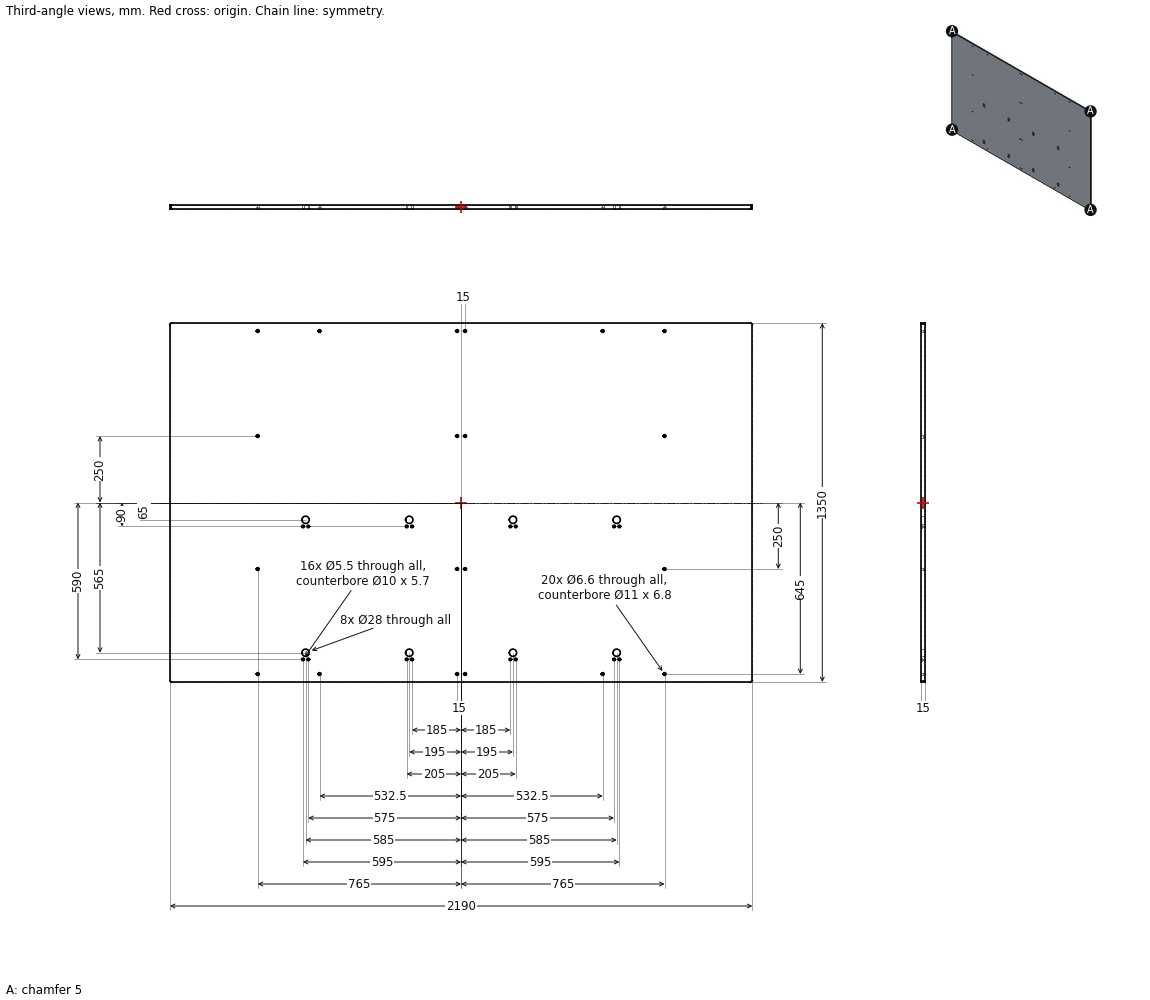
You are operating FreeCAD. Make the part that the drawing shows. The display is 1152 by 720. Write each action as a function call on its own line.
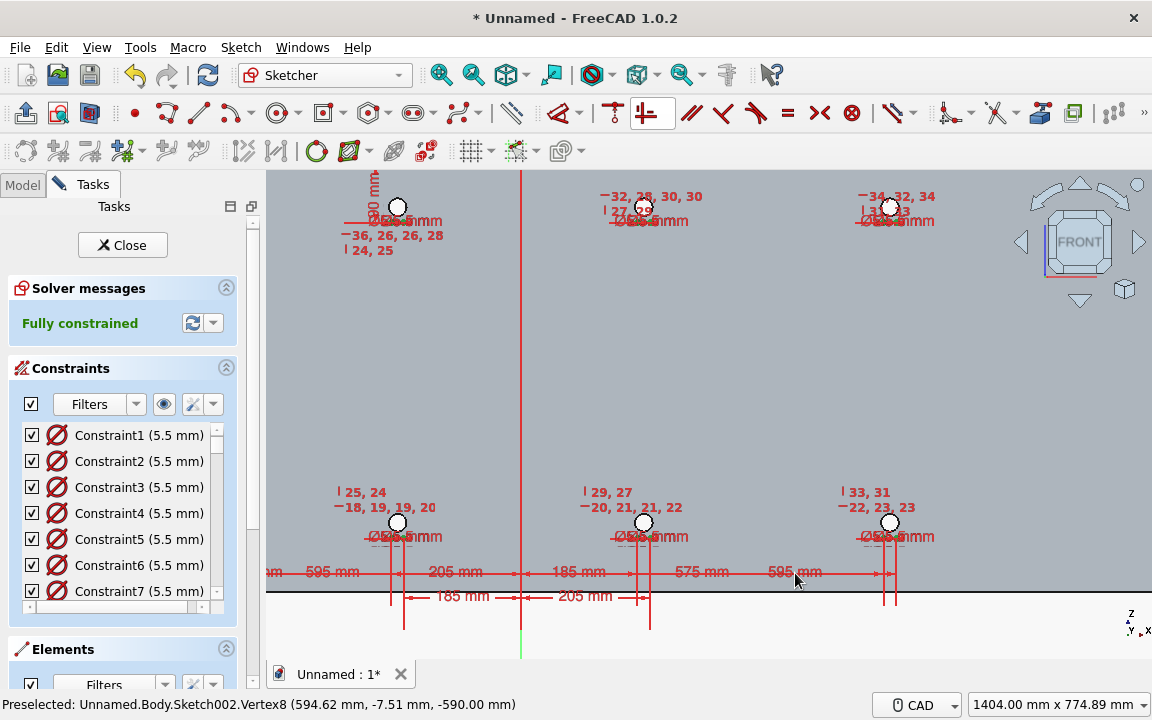
click(123, 245)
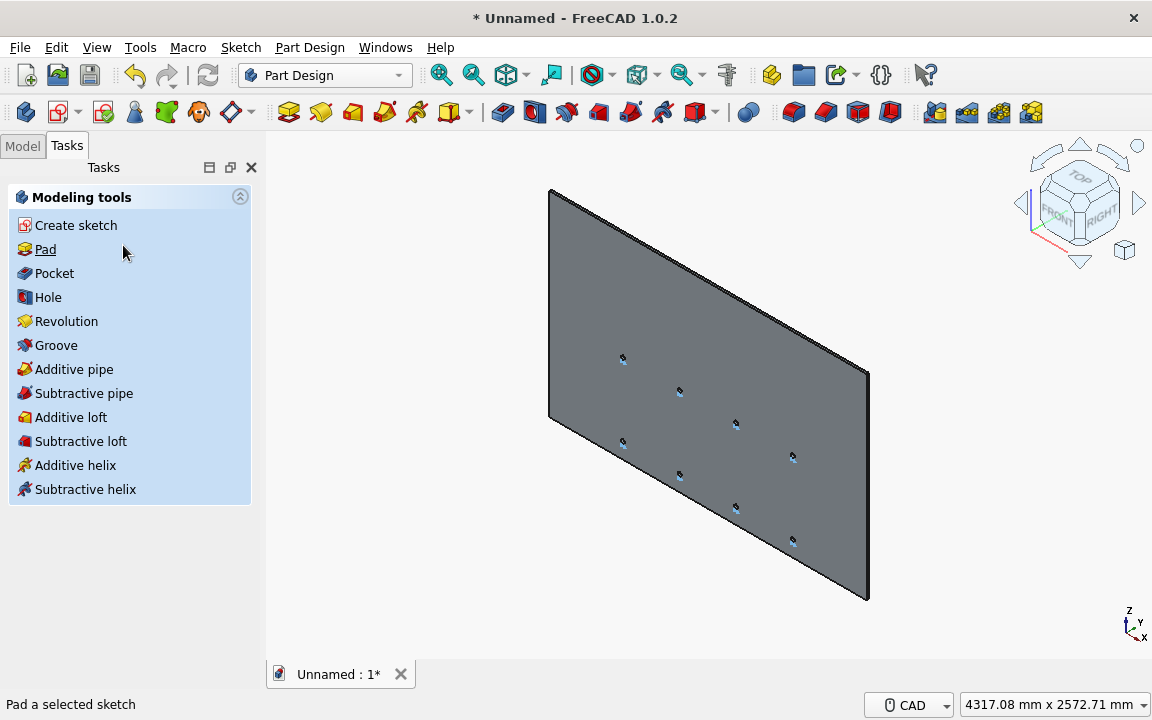
click(536, 112)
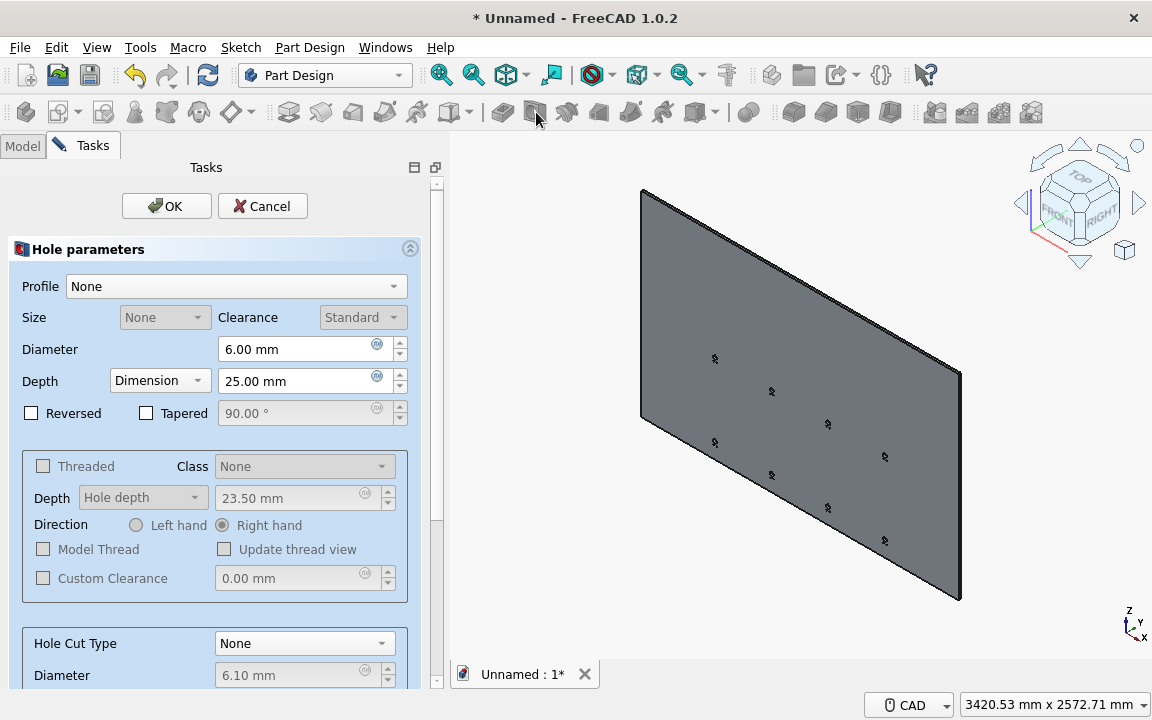
triple_click(305, 349)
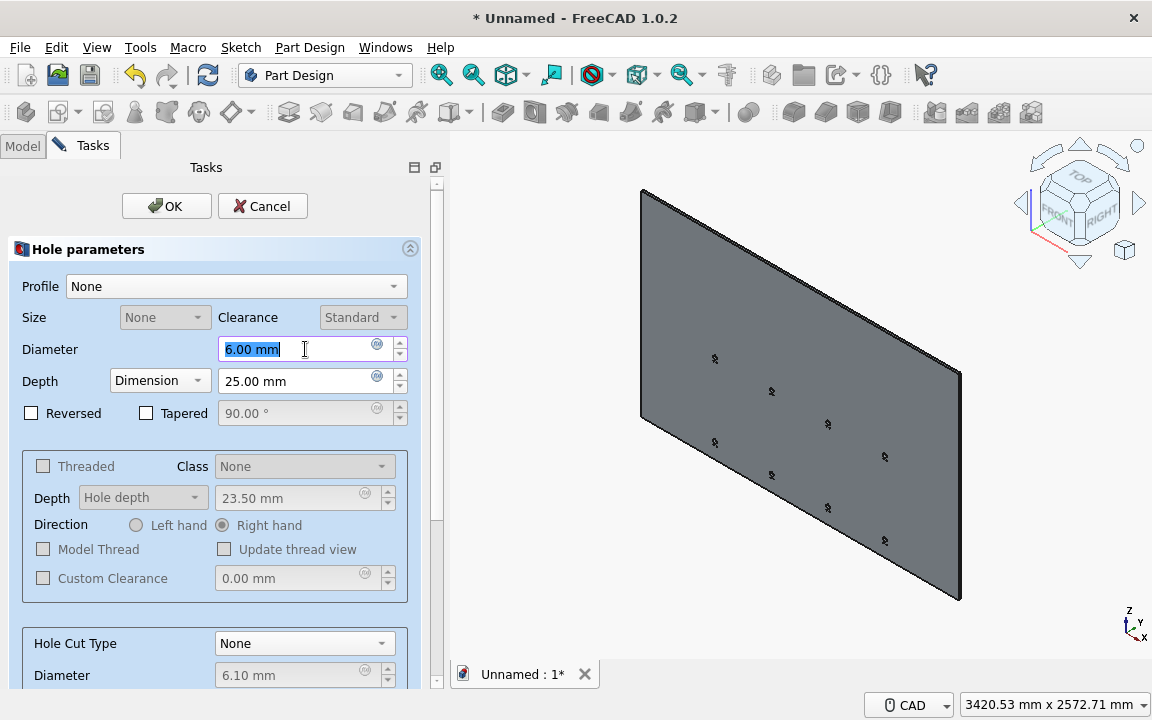
text(5.5)
key(Tab)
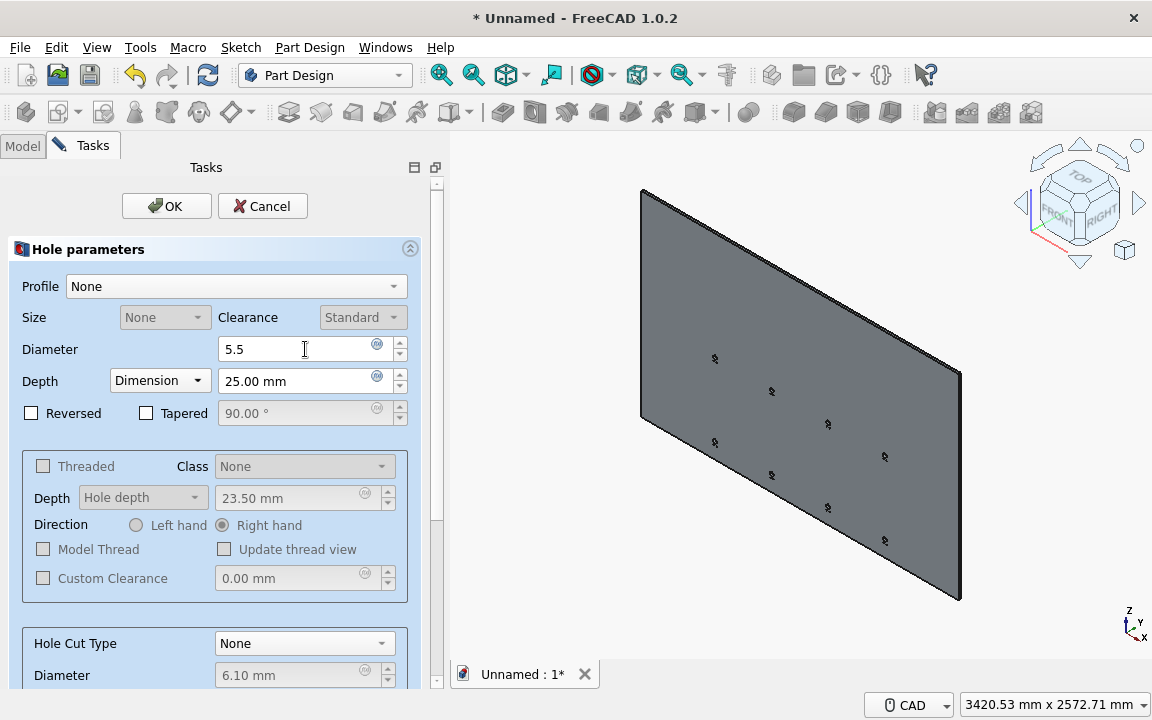
click(161, 380)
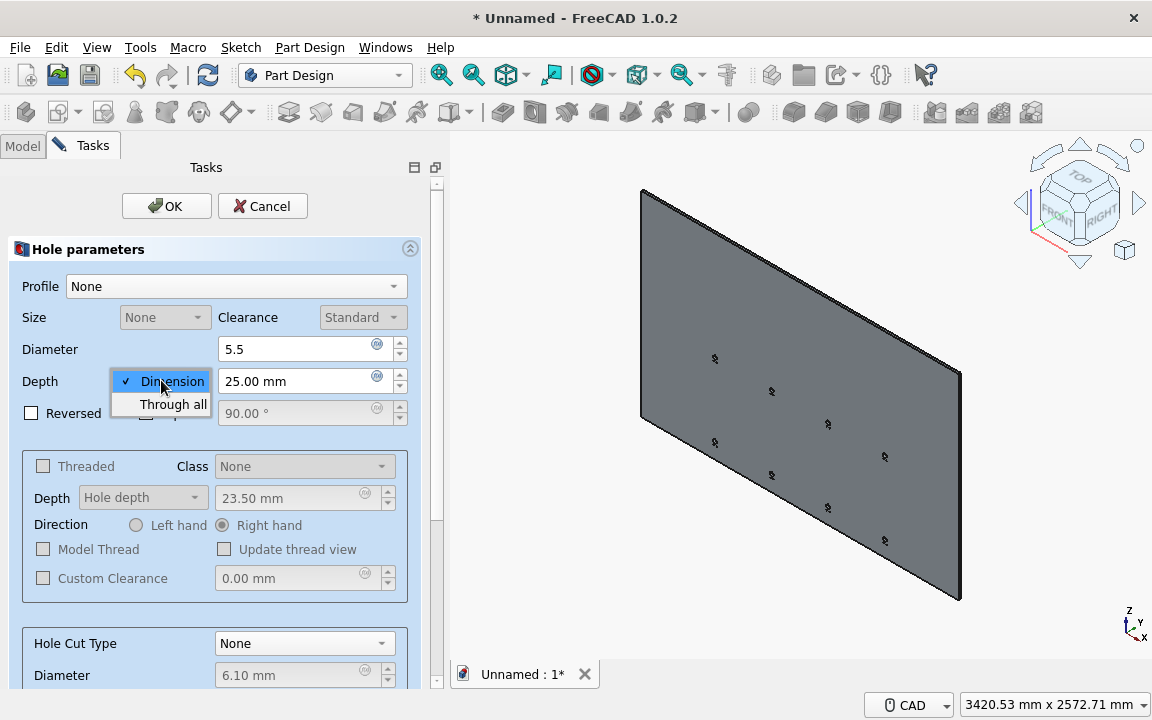
click(160, 404)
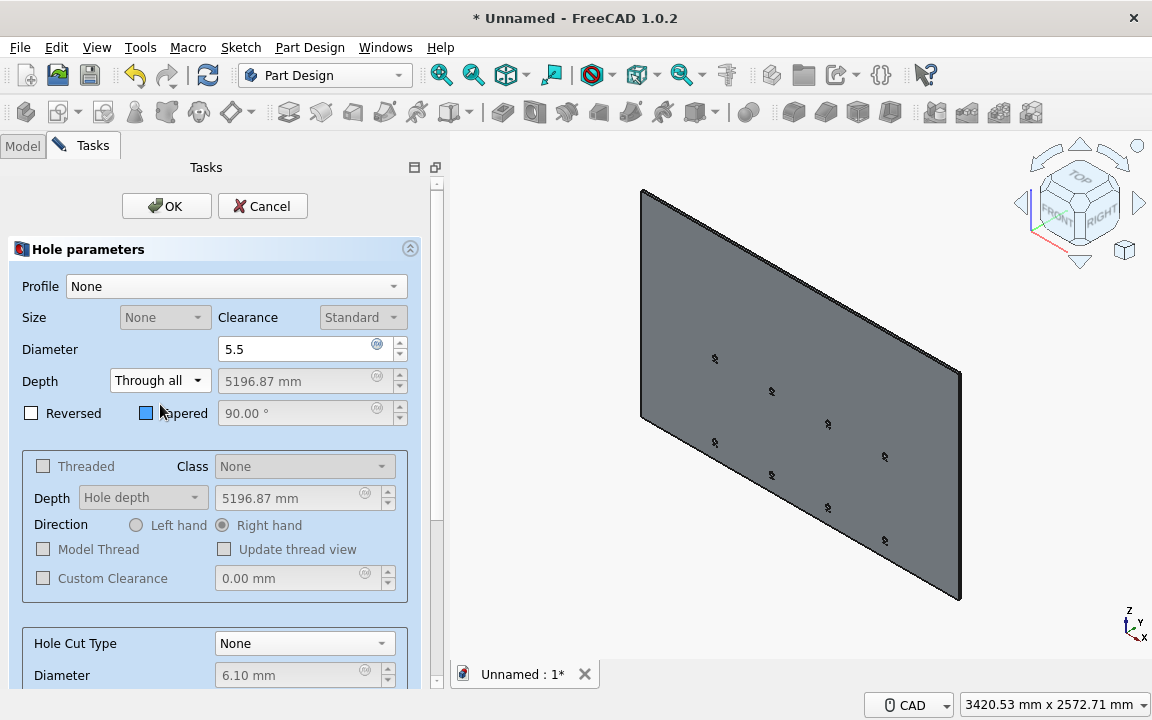
click(306, 644)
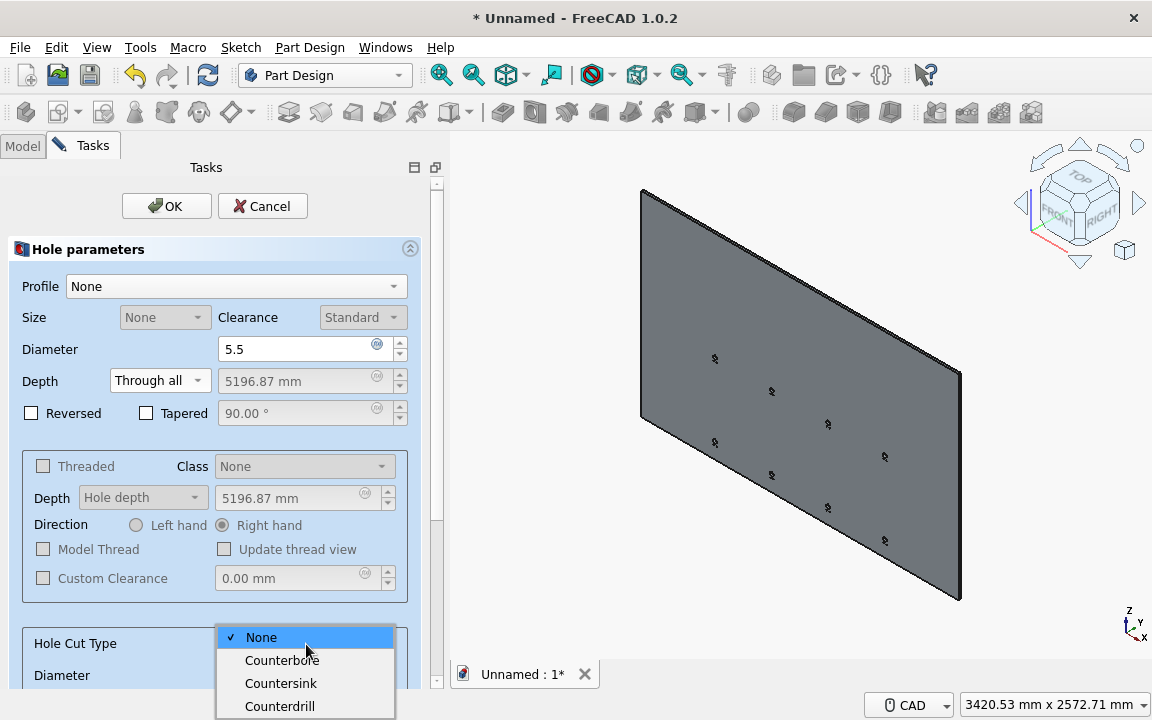
click(304, 660)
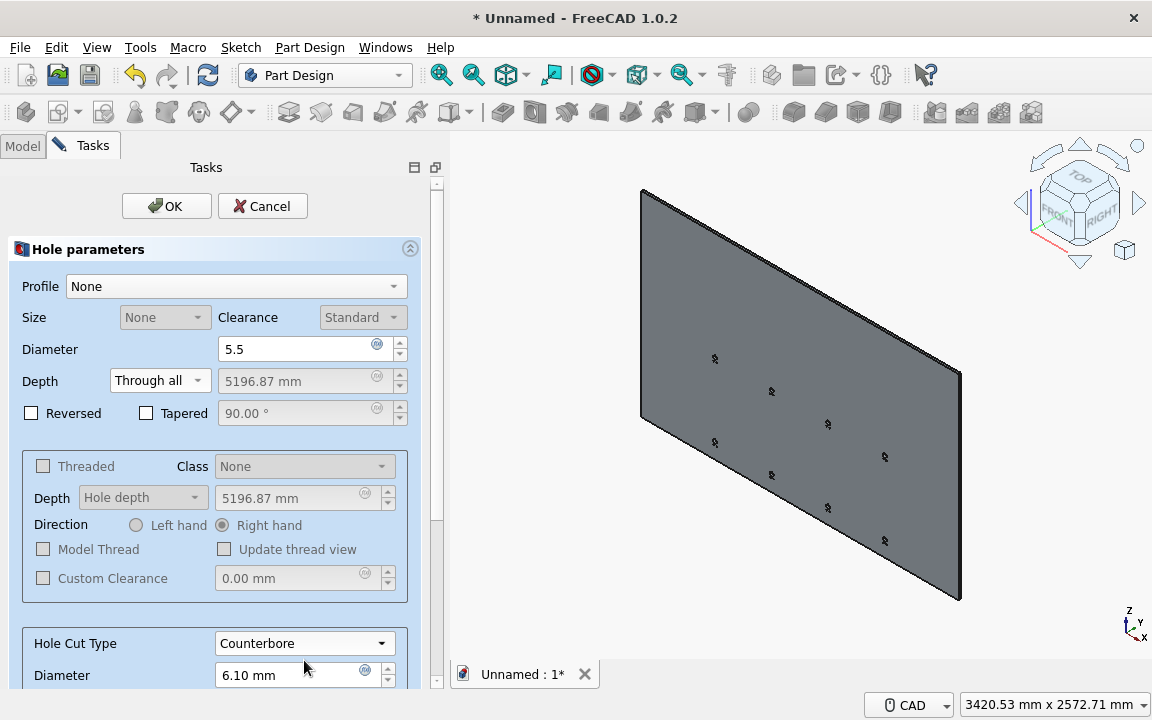
triple_click(298, 675)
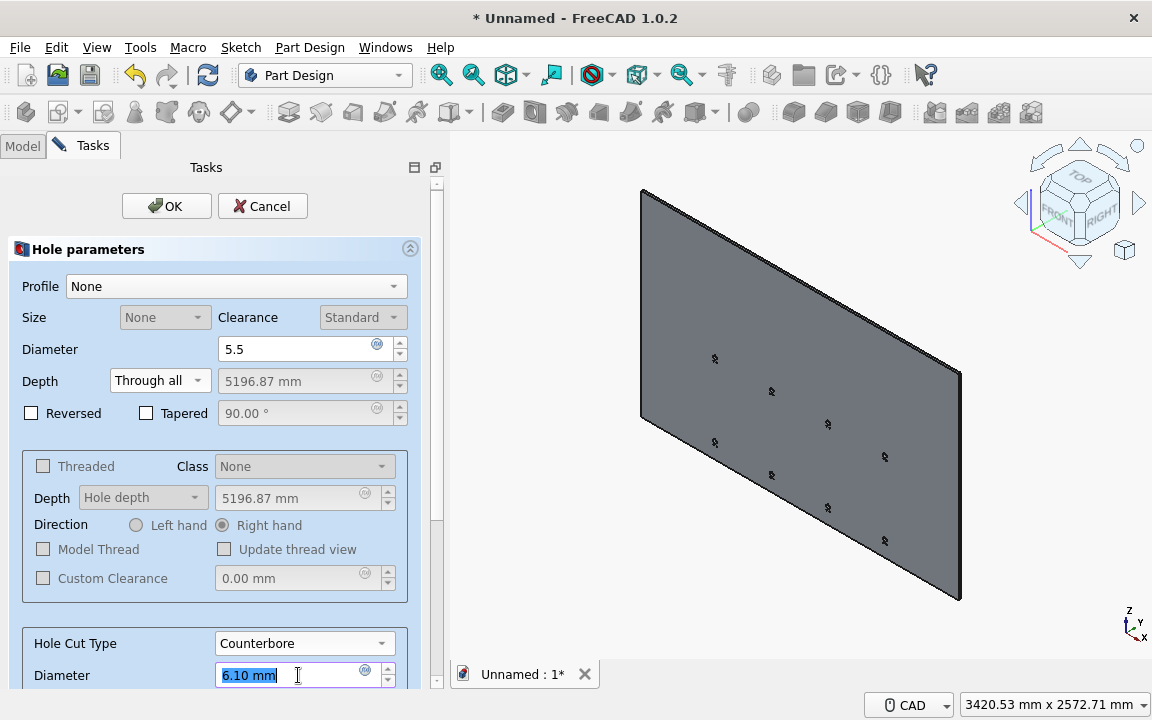
text(10)
key(Tab)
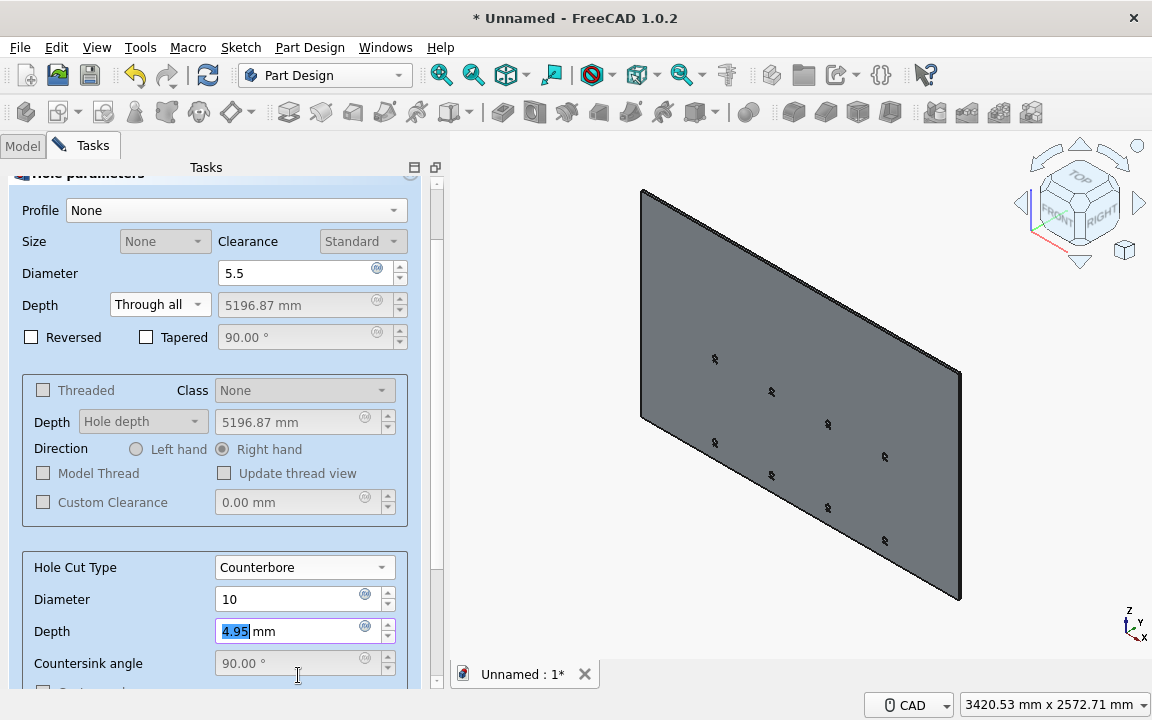
text(5.7)
key(Tab)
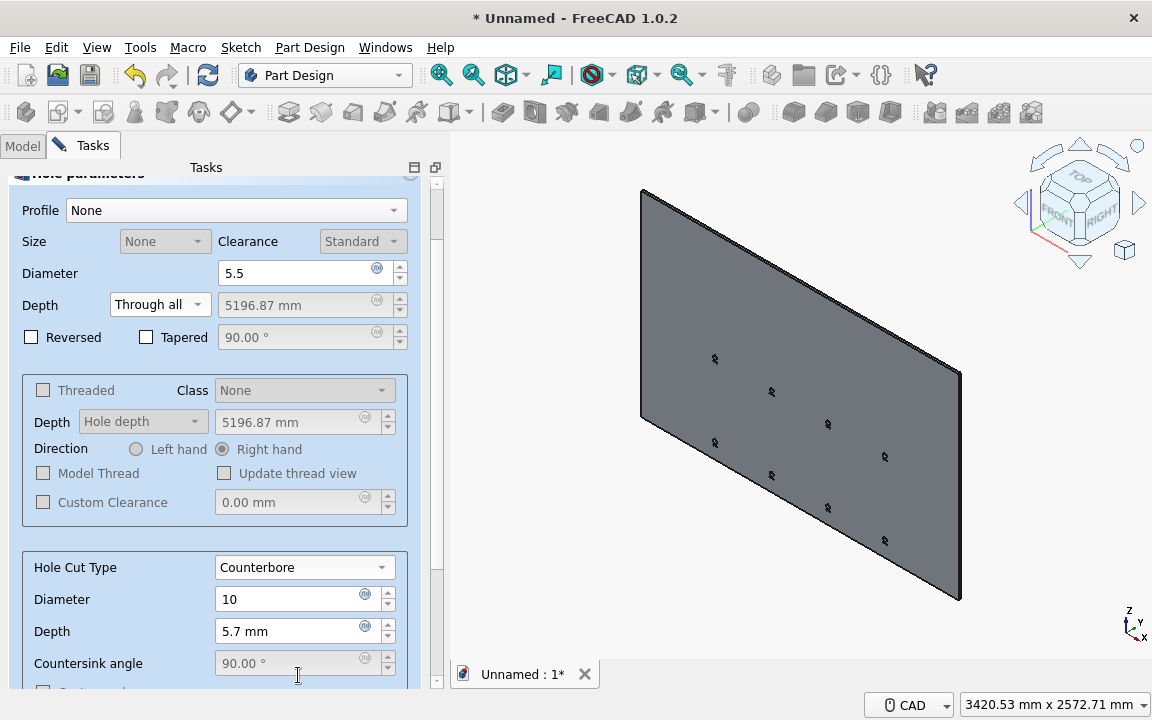
scroll(437, 432, up, 3)